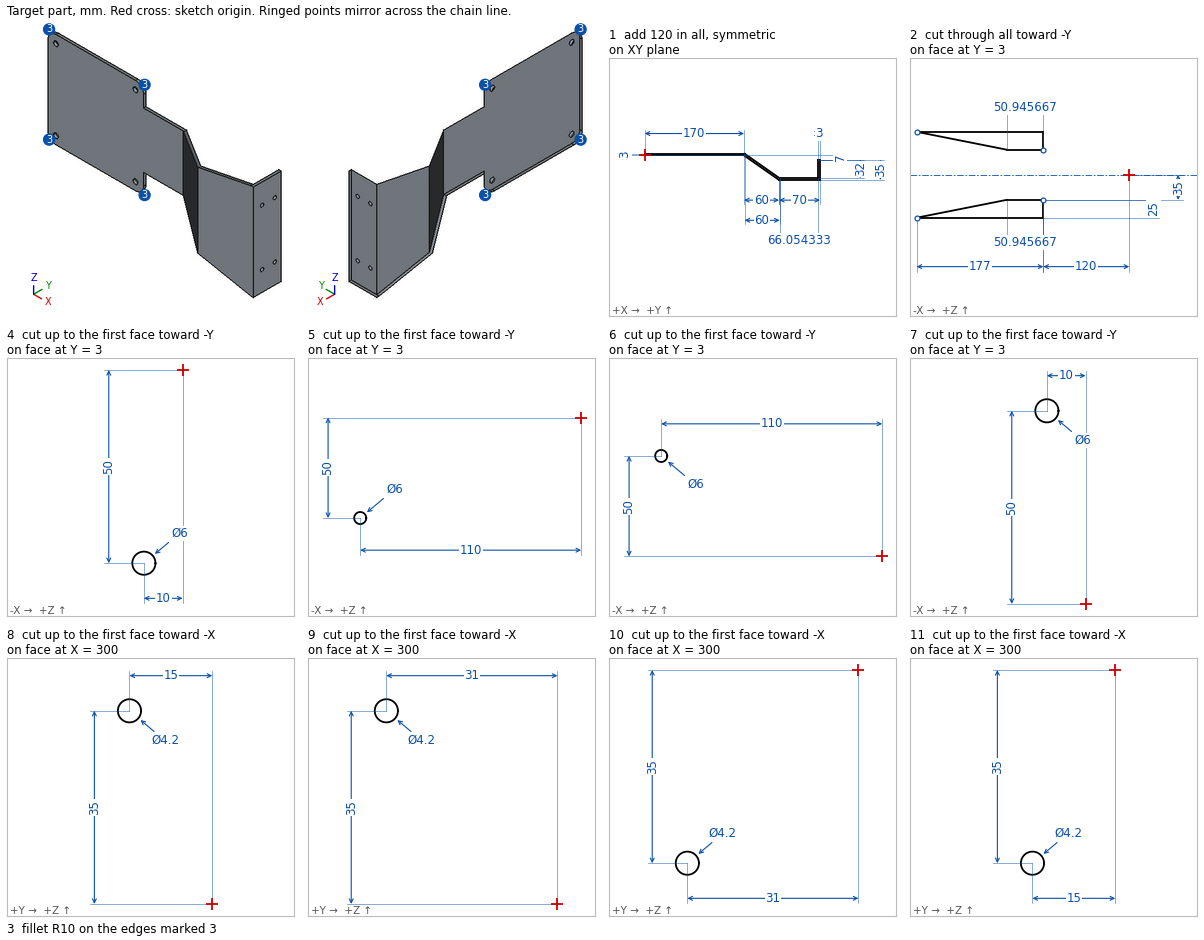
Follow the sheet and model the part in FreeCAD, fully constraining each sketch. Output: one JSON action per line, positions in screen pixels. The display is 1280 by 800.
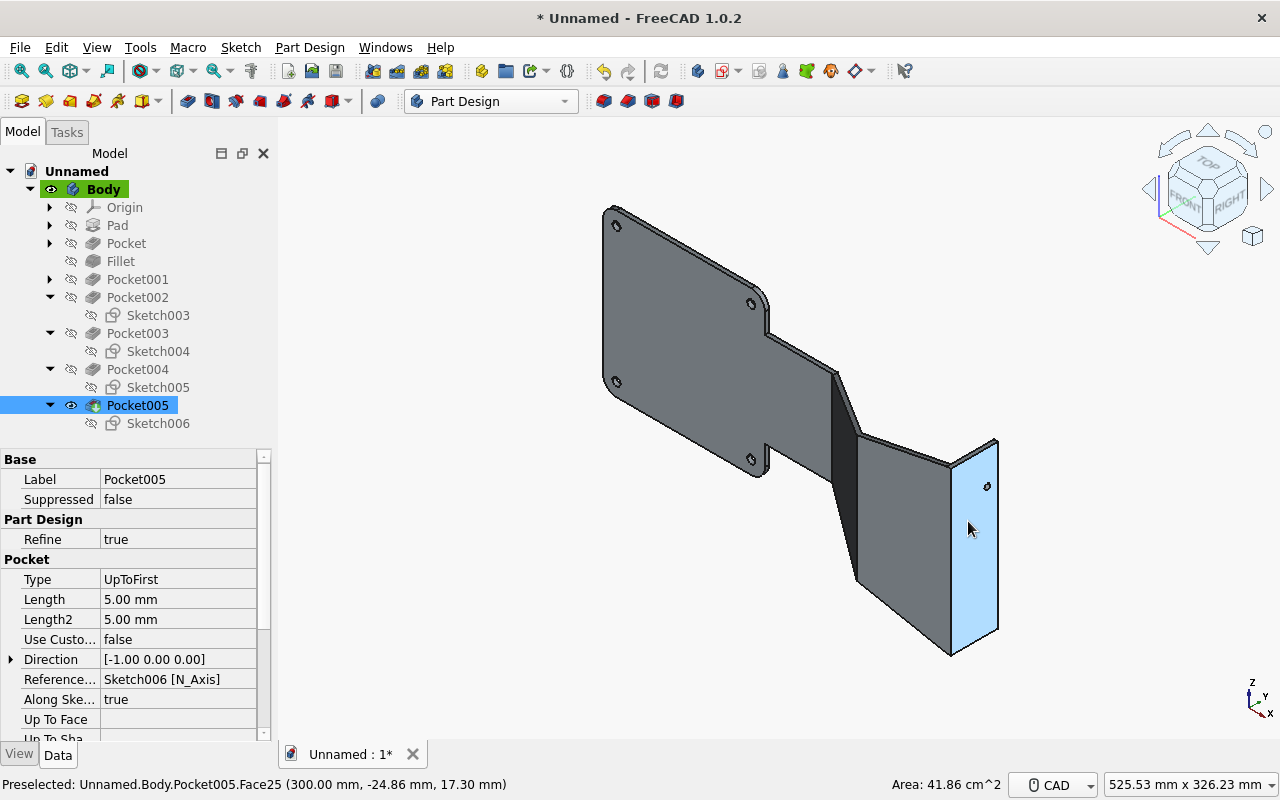
{"action": "left_click", "coordinate": [722, 72]}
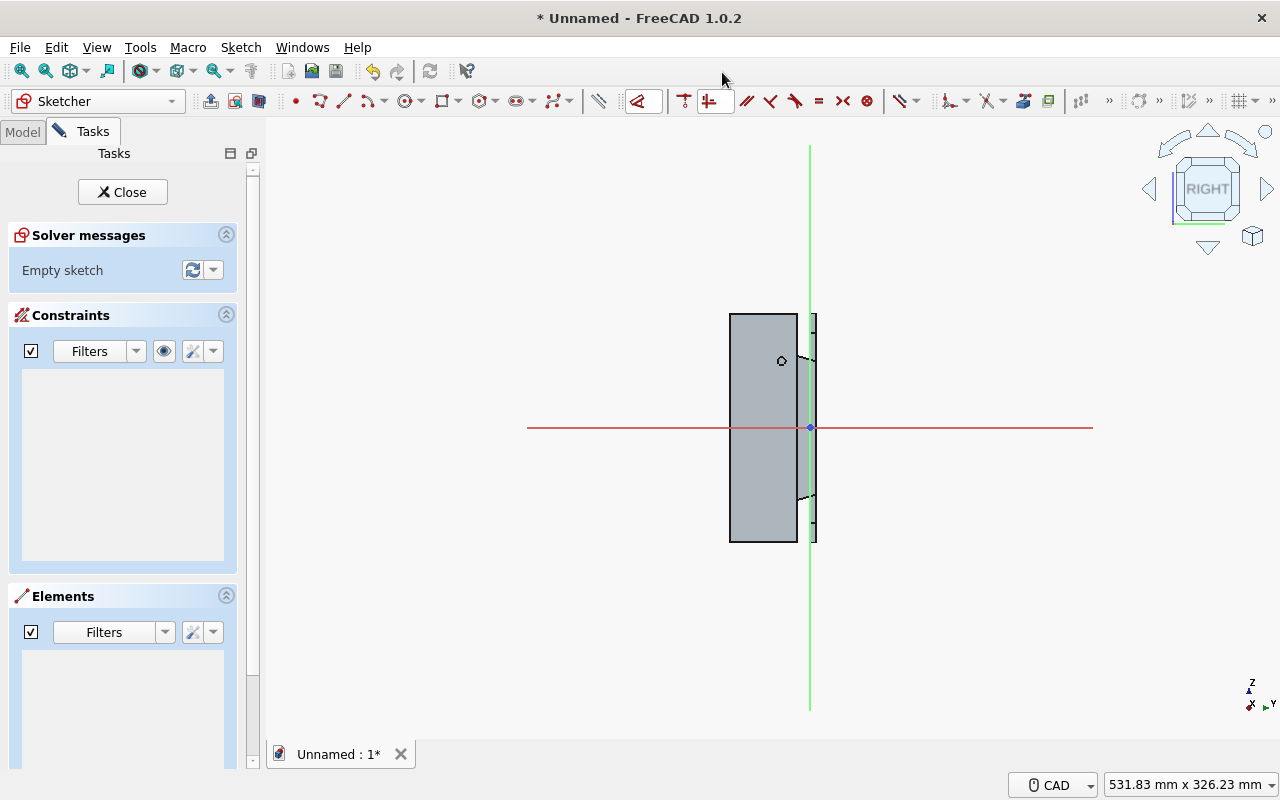
{"action": "scroll", "coordinate": [754, 358], "scroll_direction": "up", "scroll_amount": 15}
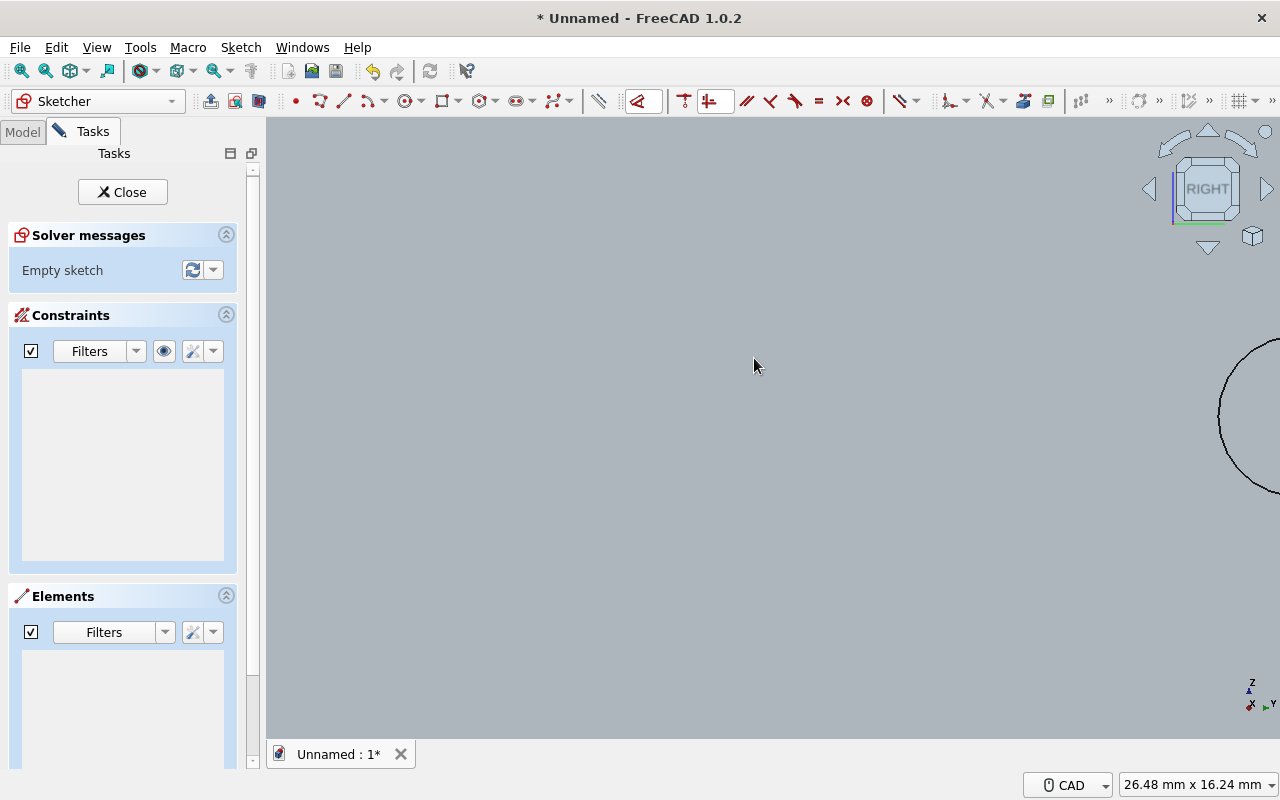
{"action": "scroll", "coordinate": [675, 409], "scroll_direction": "up", "scroll_amount": 5}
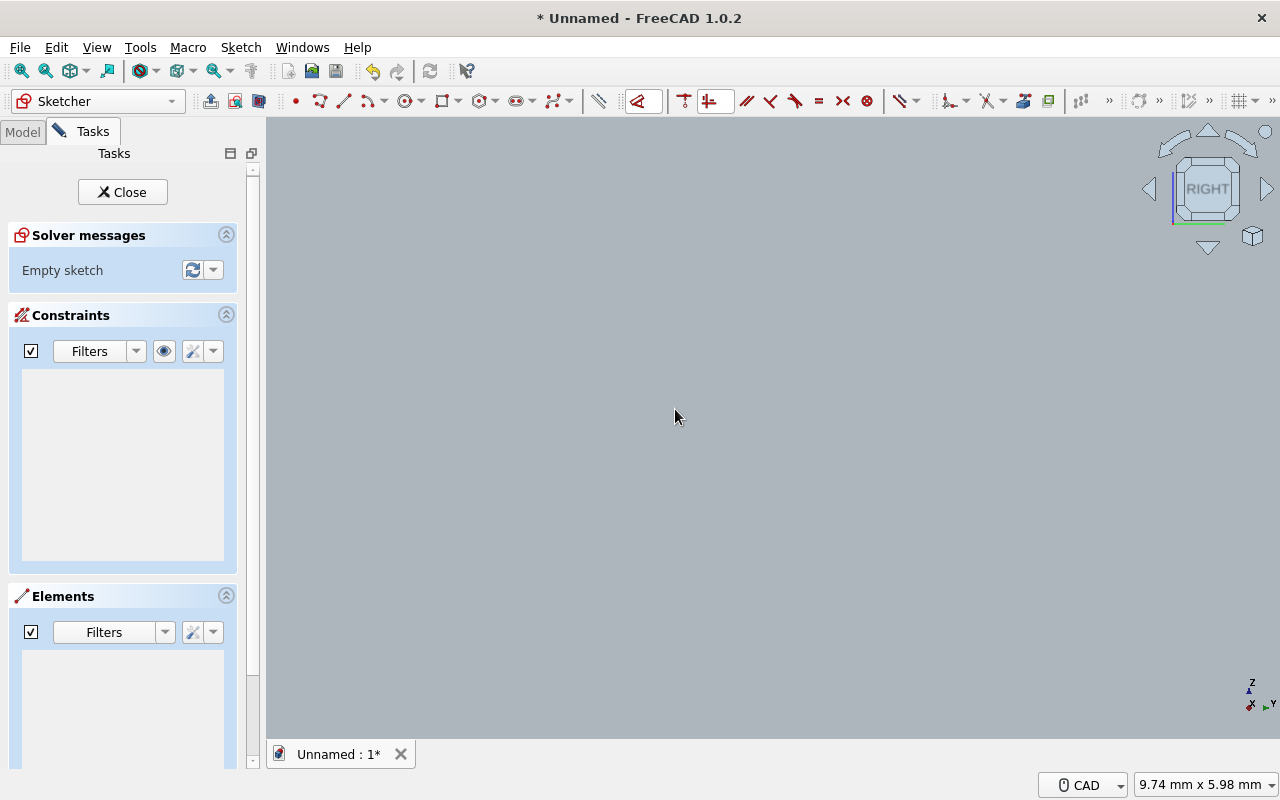
{"action": "left_click", "coordinate": [406, 102]}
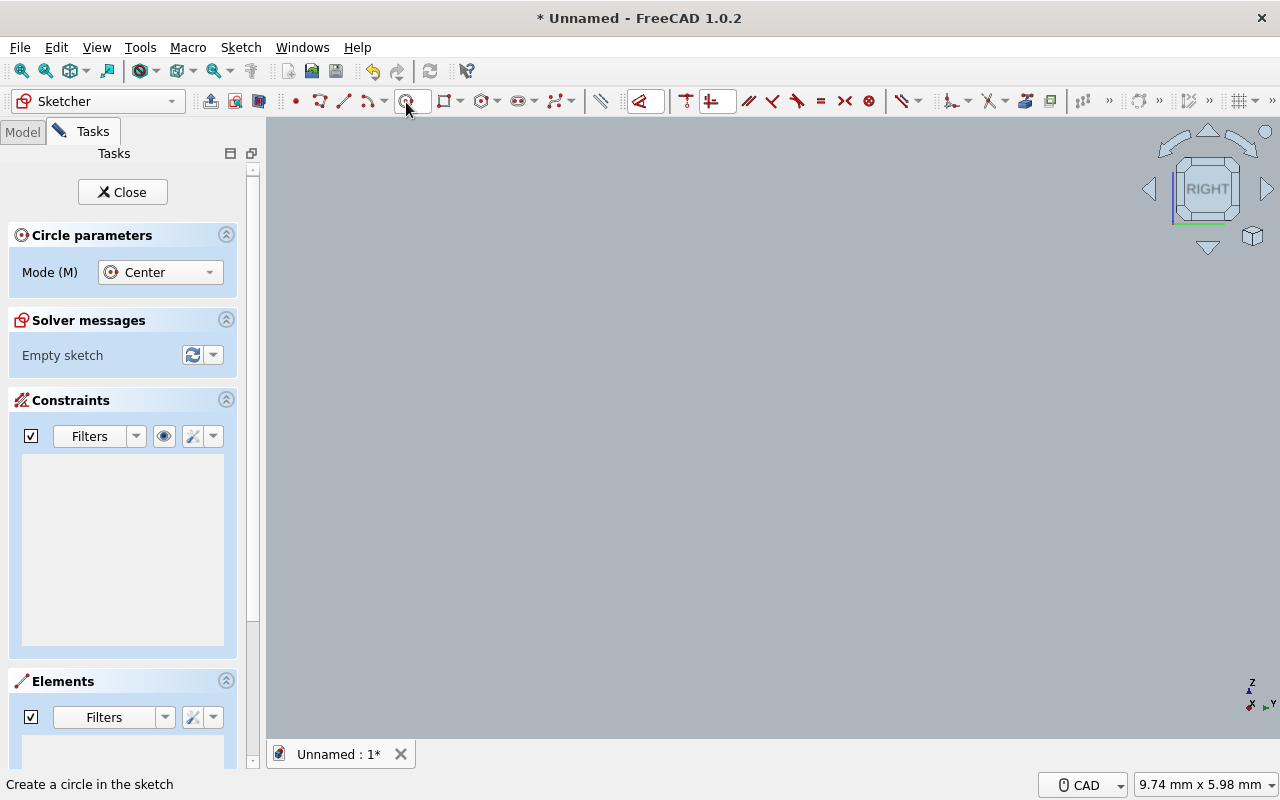
{"action": "left_click", "coordinate": [704, 428]}
{"action": "left_click", "coordinate": [859, 273]}
{"action": "key", "text": "Escape"}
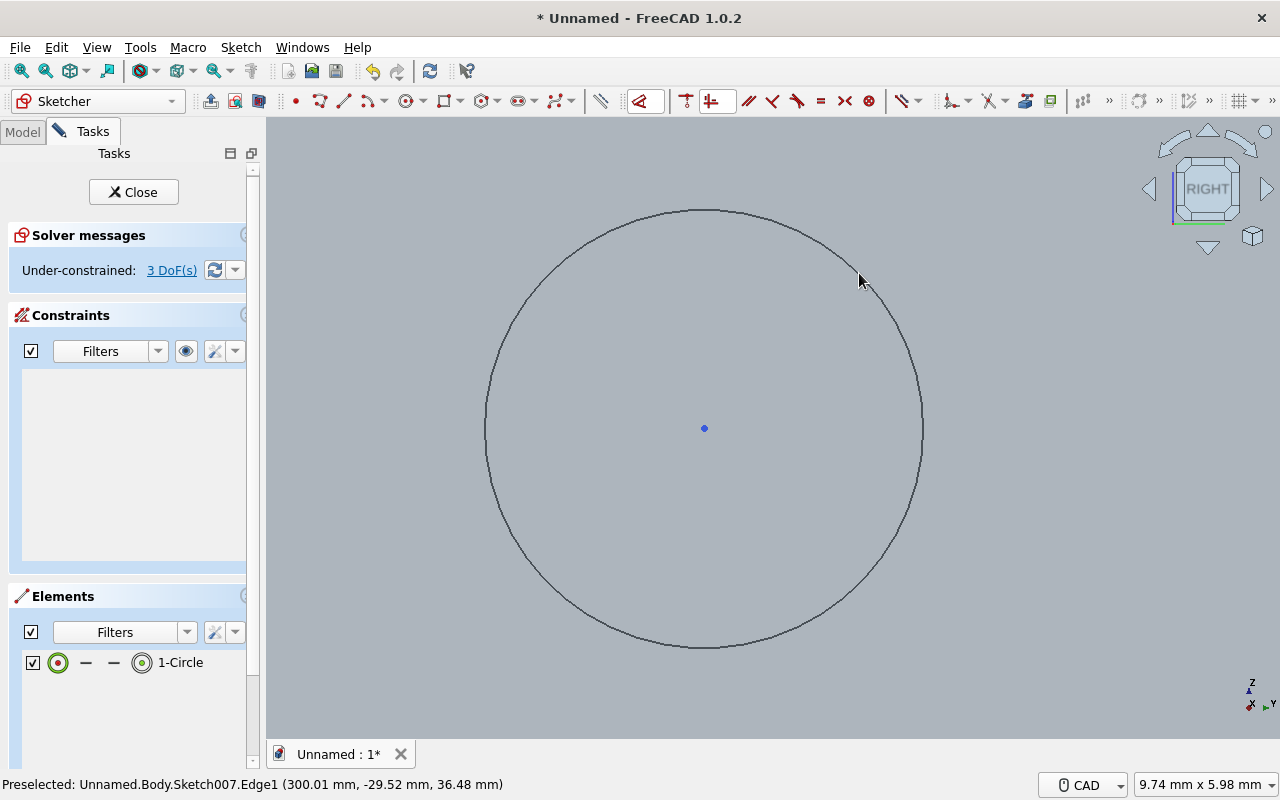
{"action": "left_click", "coordinate": [859, 274]}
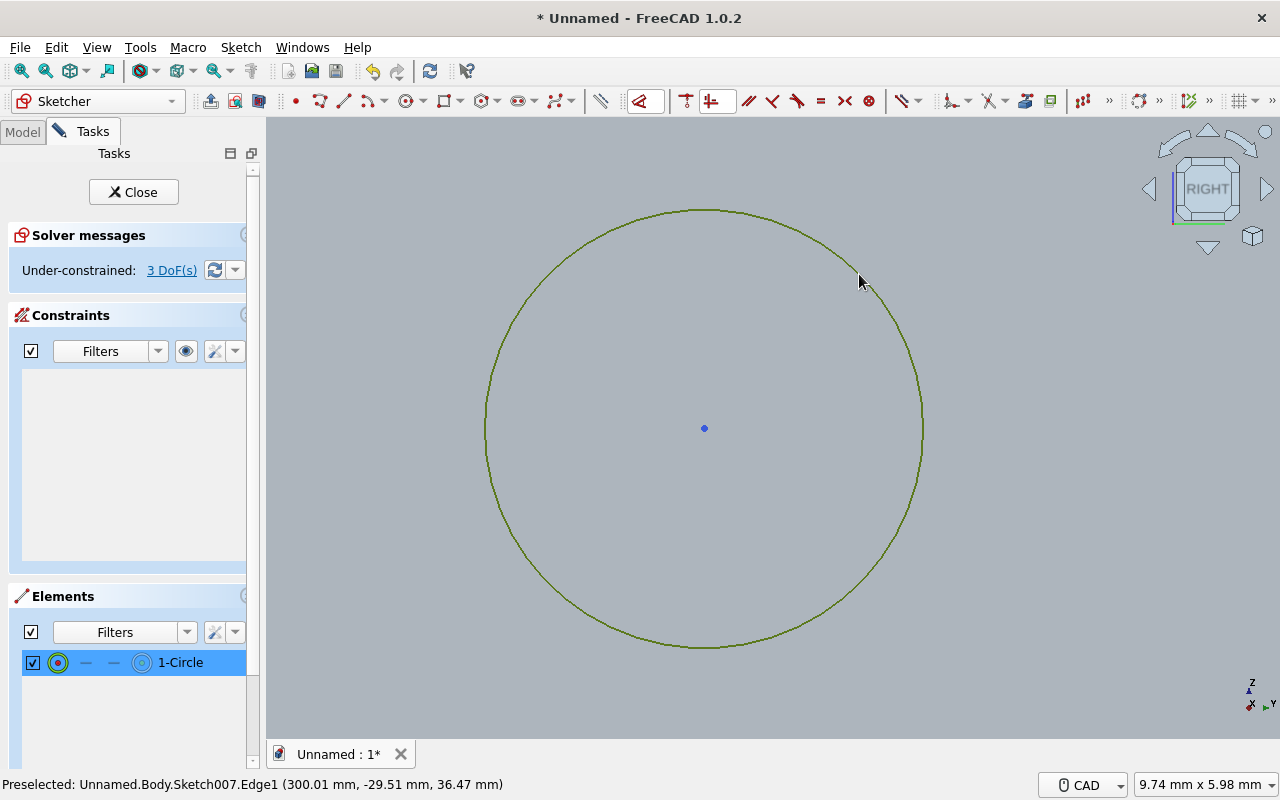
{"action": "left_click", "coordinate": [658, 102]}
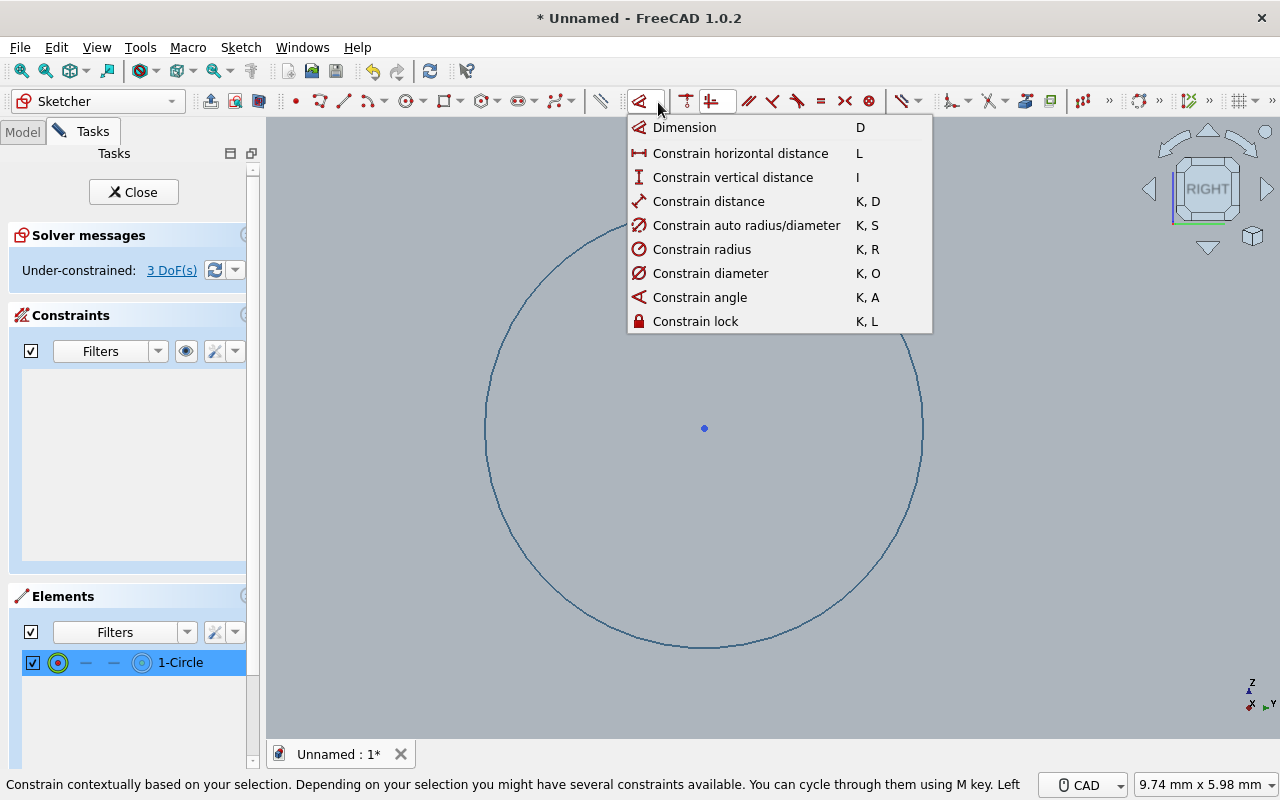
{"action": "left_click", "coordinate": [780, 273]}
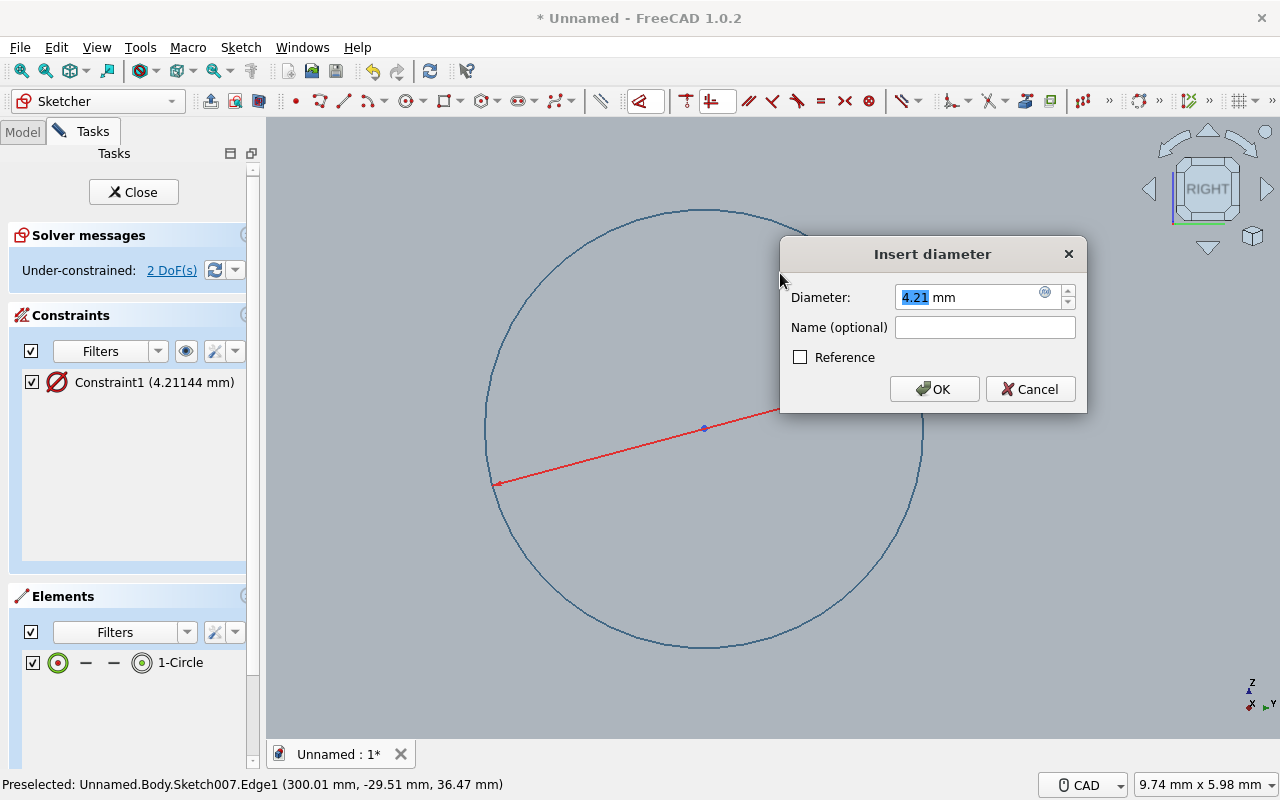
{"action": "type", "text": "4.2"}
{"action": "key", "text": "Return"}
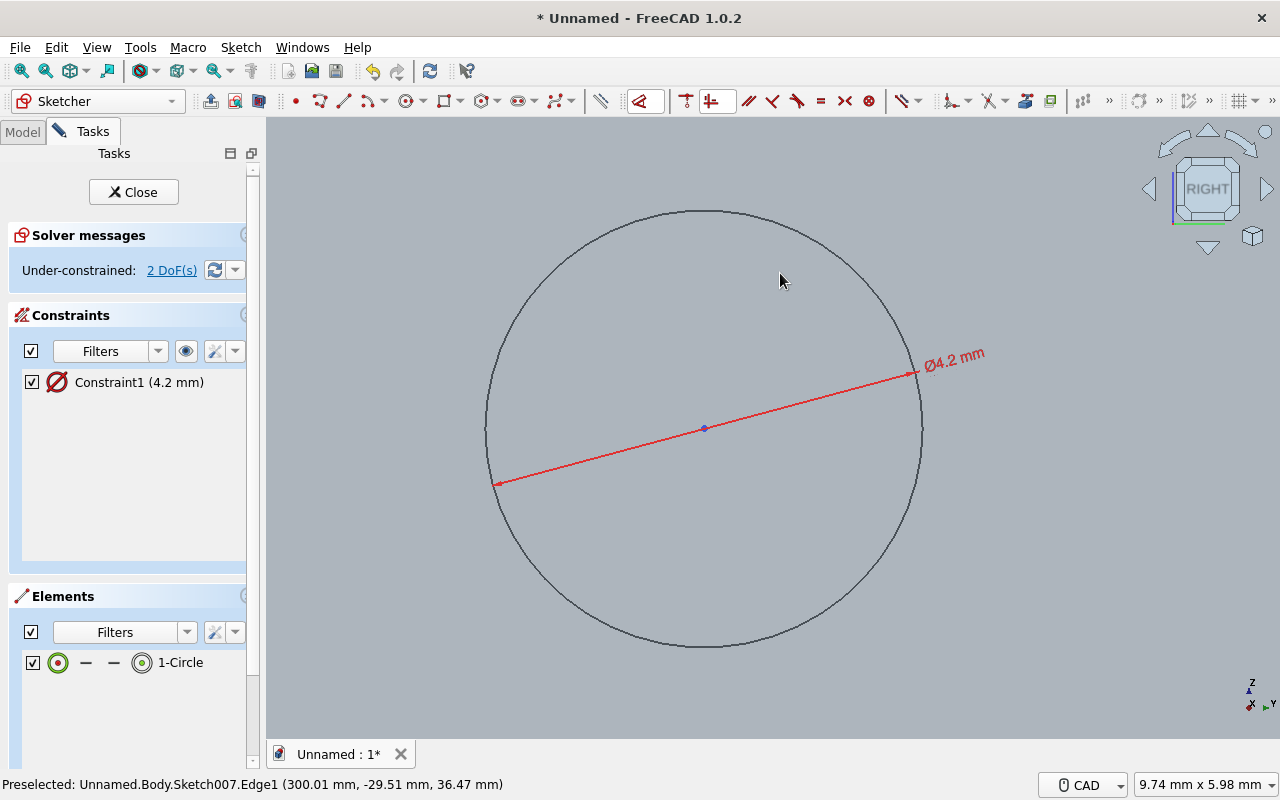
{"action": "left_click", "coordinate": [704, 429]}